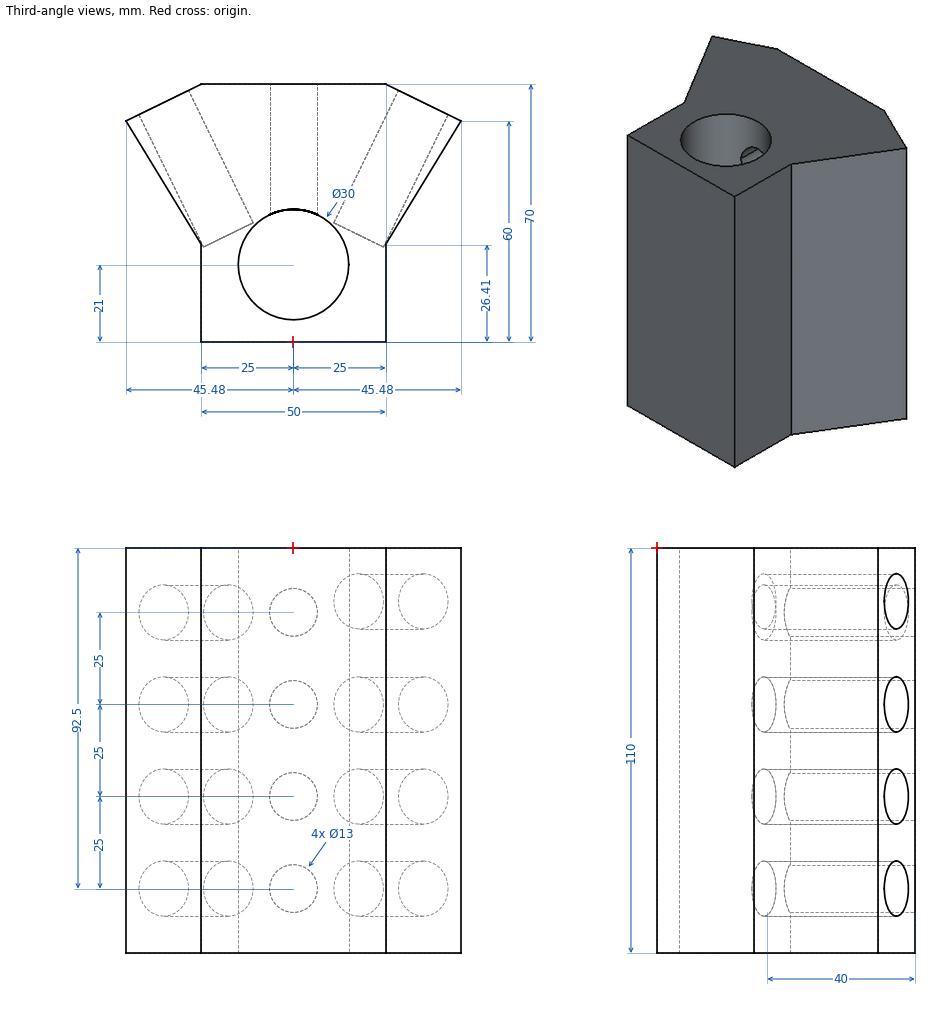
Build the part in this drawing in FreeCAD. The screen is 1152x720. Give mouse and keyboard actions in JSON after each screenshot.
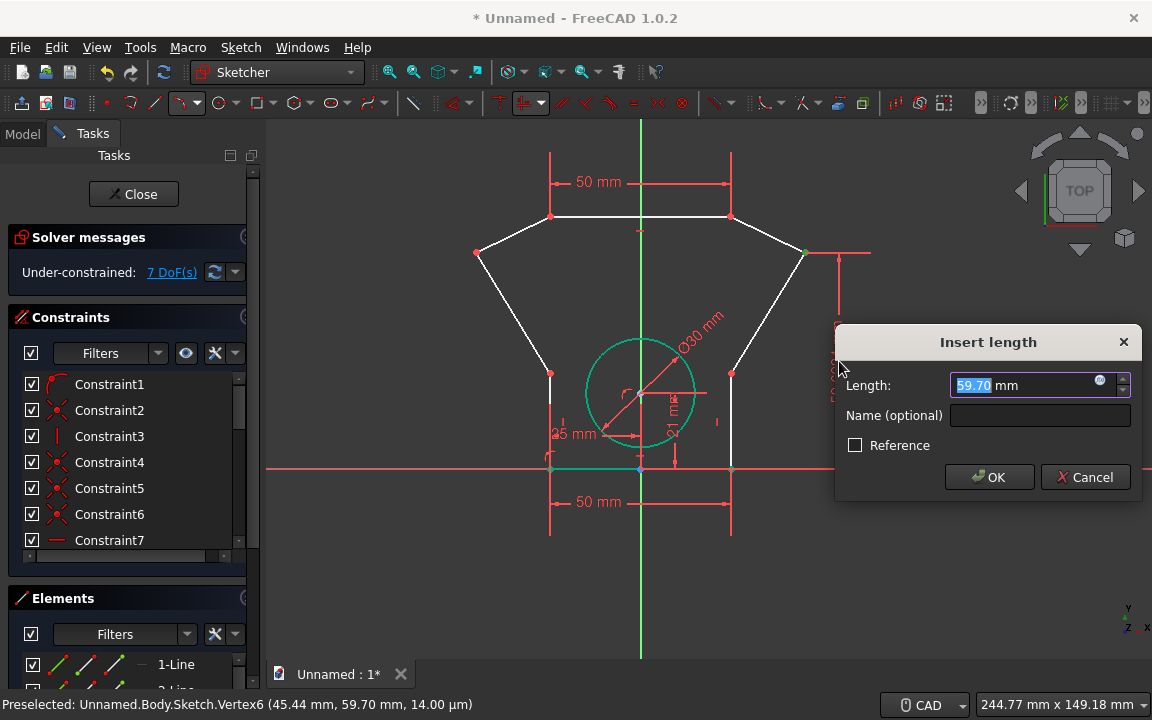
{"action": "type", "text": "60"}
{"action": "key", "text": "Return"}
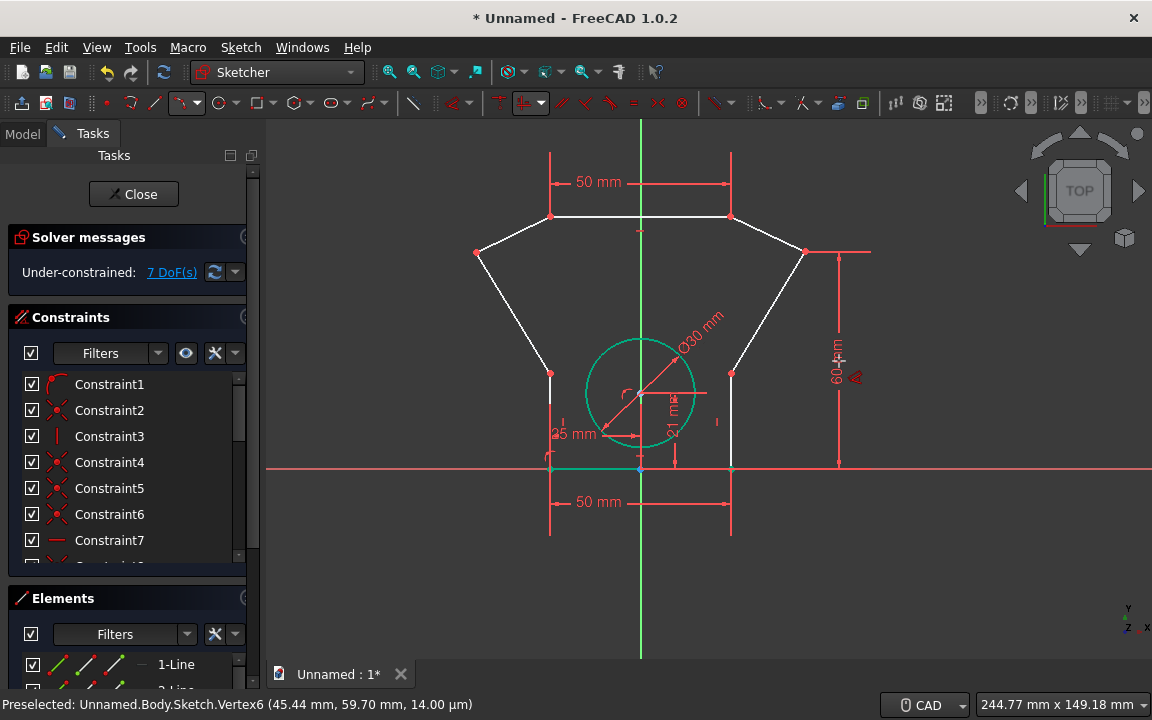
{"action": "left_click", "coordinate": [731, 217]}
{"action": "left_click", "coordinate": [686, 503]}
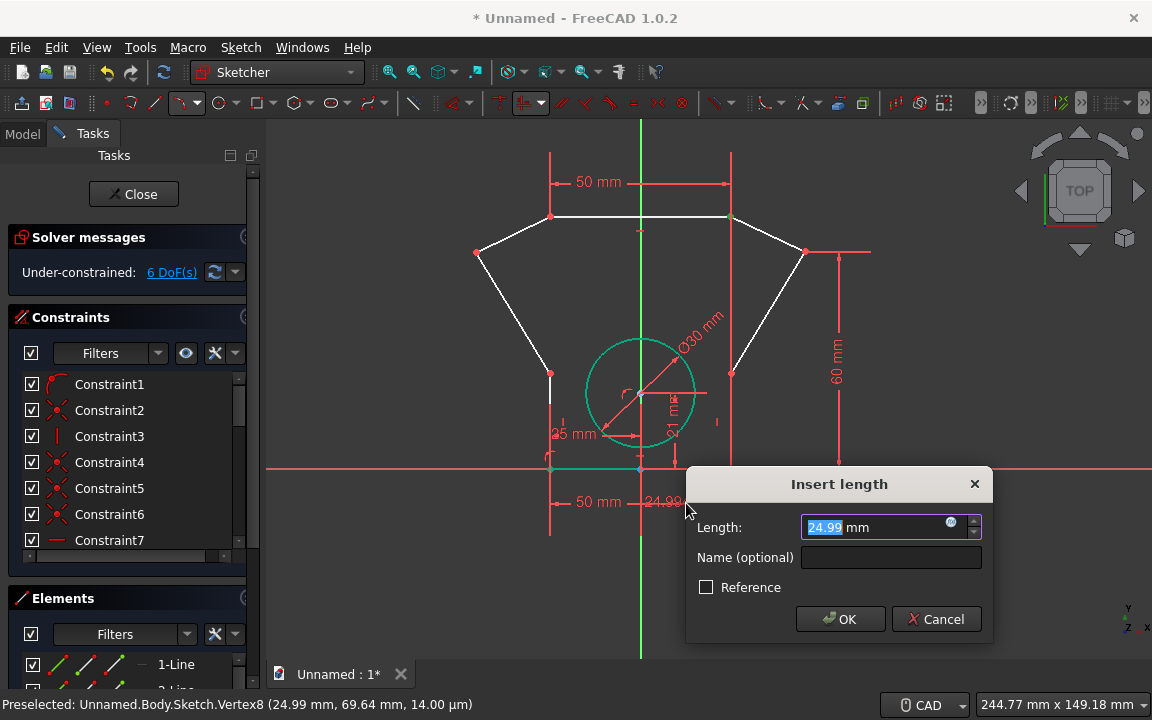
{"action": "type", "text": "25"}
{"action": "key", "text": "Return"}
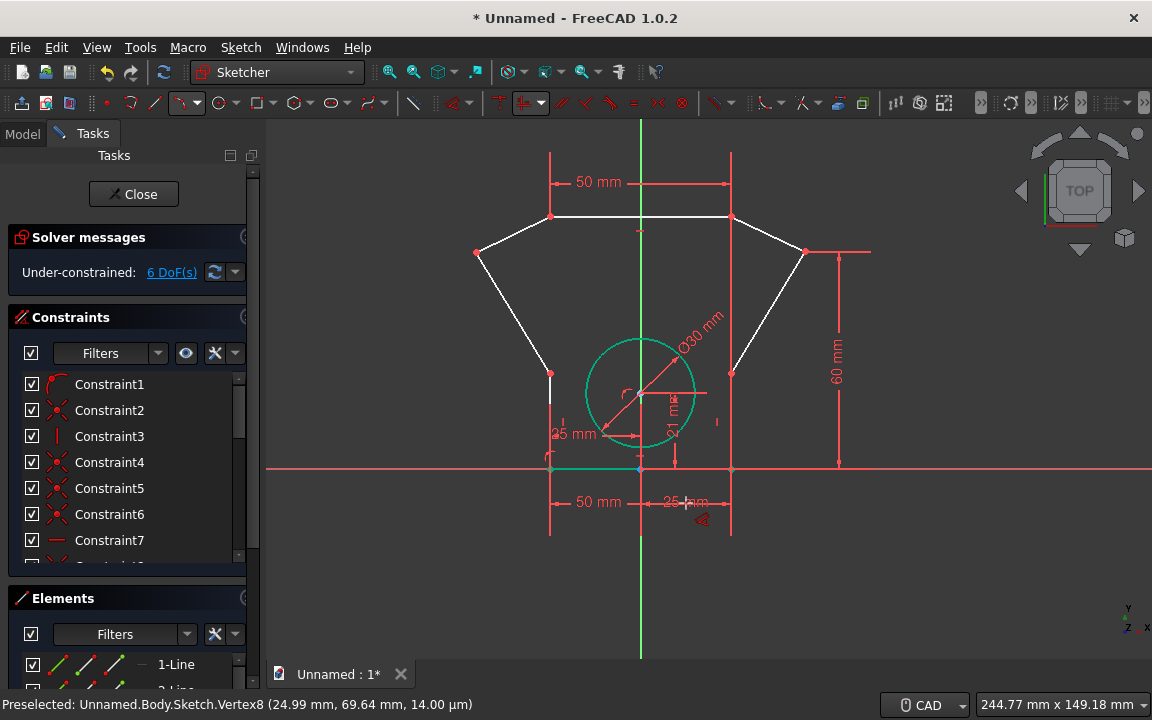
{"action": "left_click", "coordinate": [731, 217]}
{"action": "left_click", "coordinate": [765, 285]}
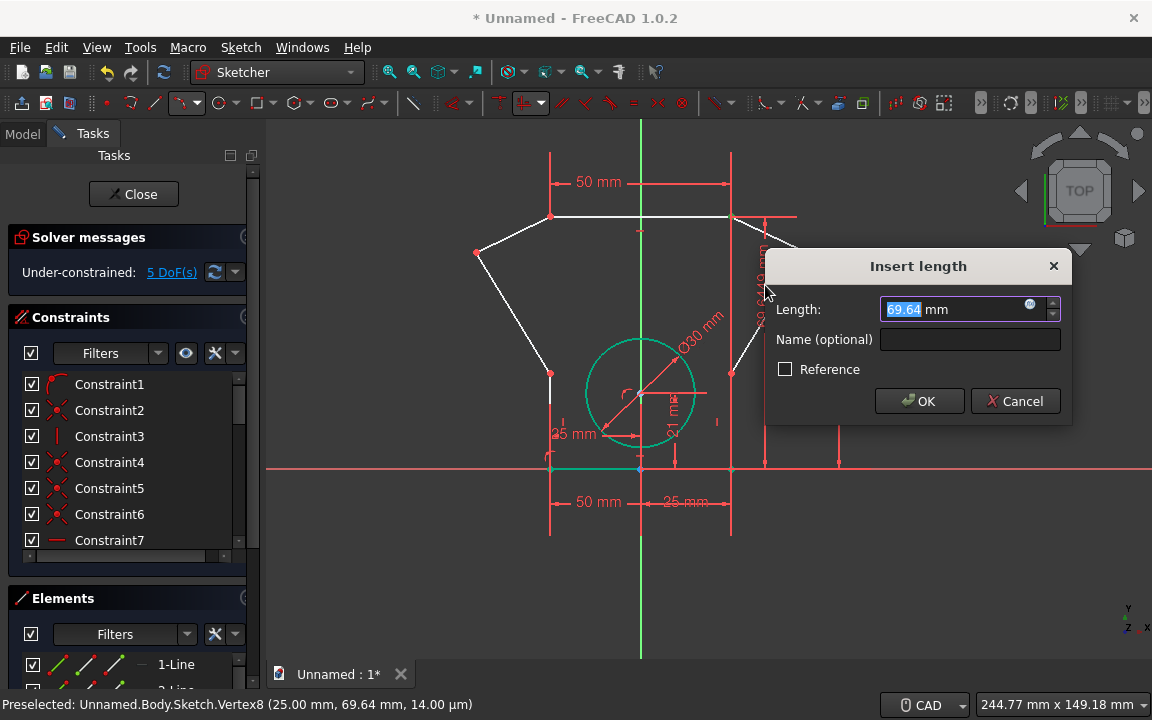
{"action": "type", "text": "70"}
{"action": "key", "text": "Return"}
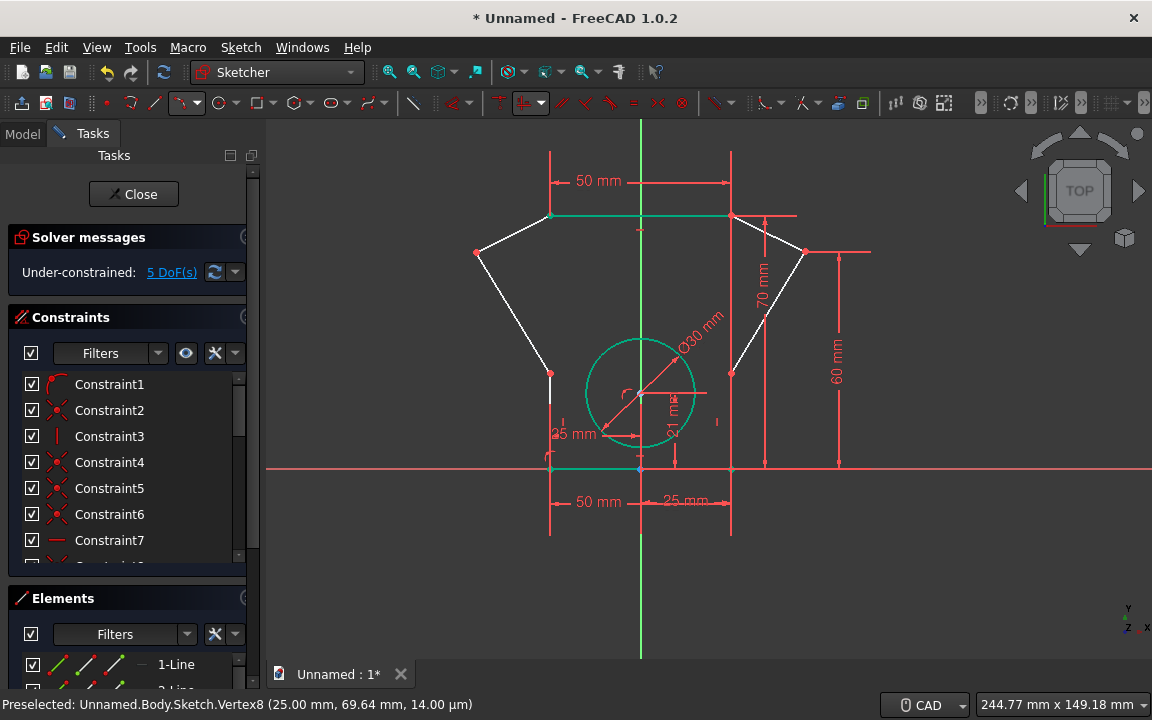
{"action": "left_click", "coordinate": [476, 253]}
{"action": "left_click", "coordinate": [442, 361]}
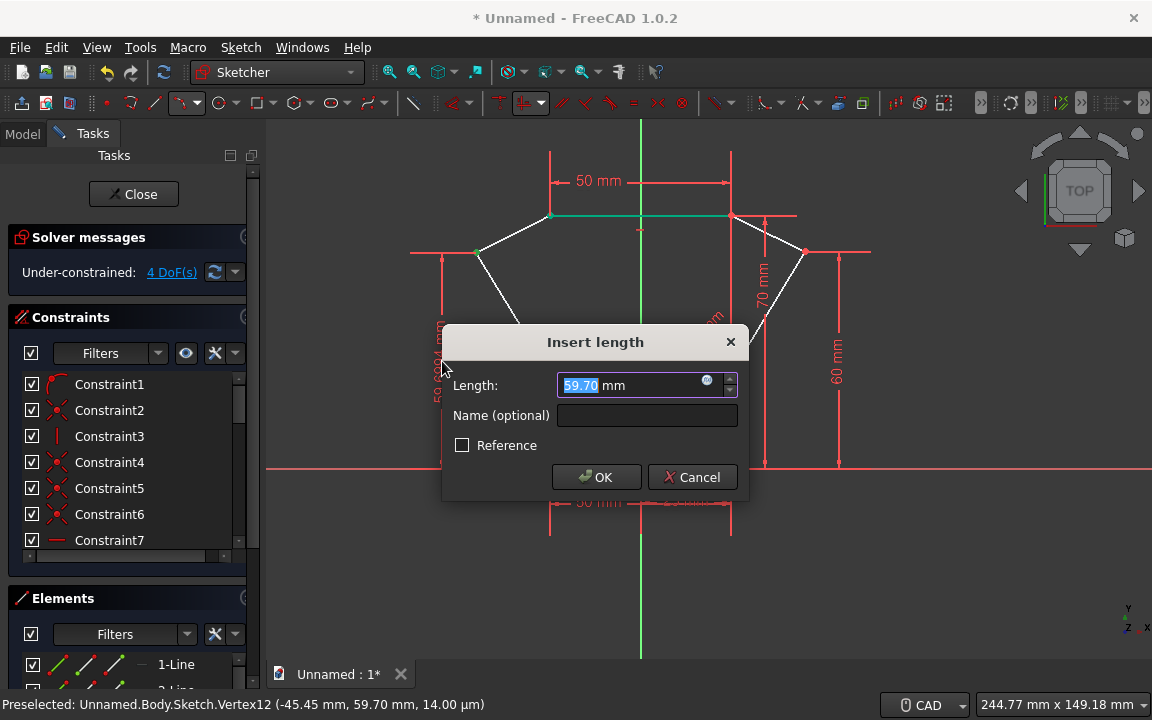
{"action": "type", "text": "60"}
{"action": "key", "text": "Return"}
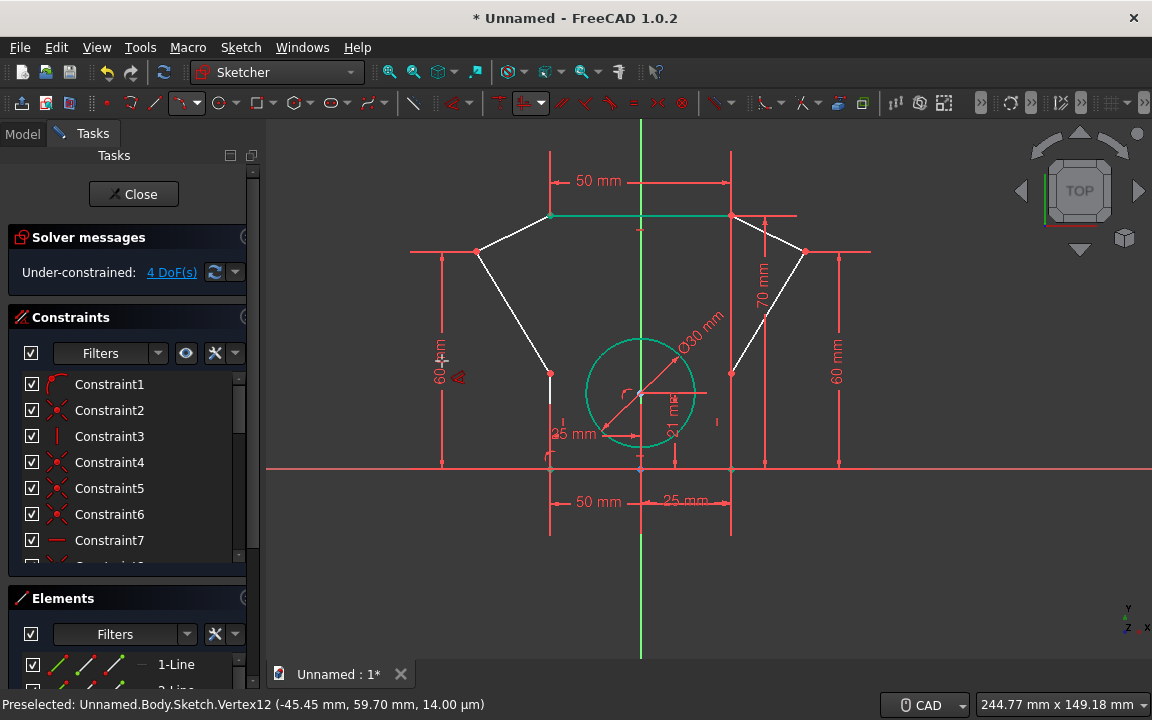
{"action": "left_click", "coordinate": [731, 441]}
{"action": "left_click", "coordinate": [765, 422]}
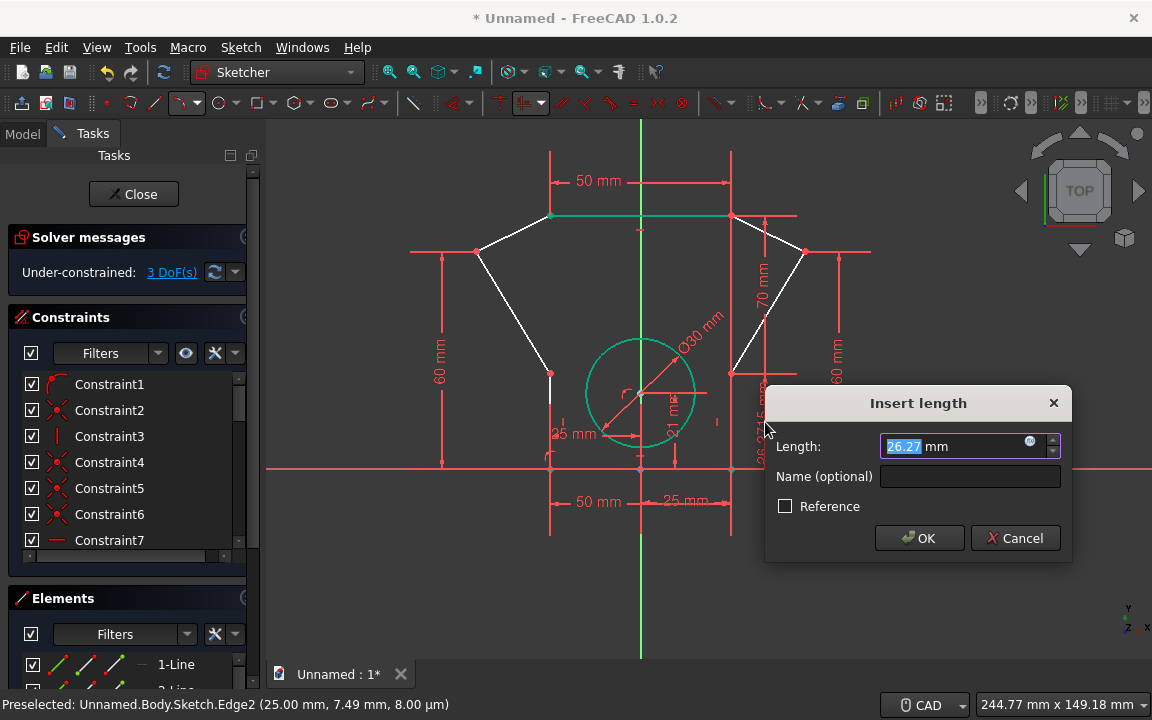
{"action": "type", "text": "26.41"}
{"action": "key", "text": "Return"}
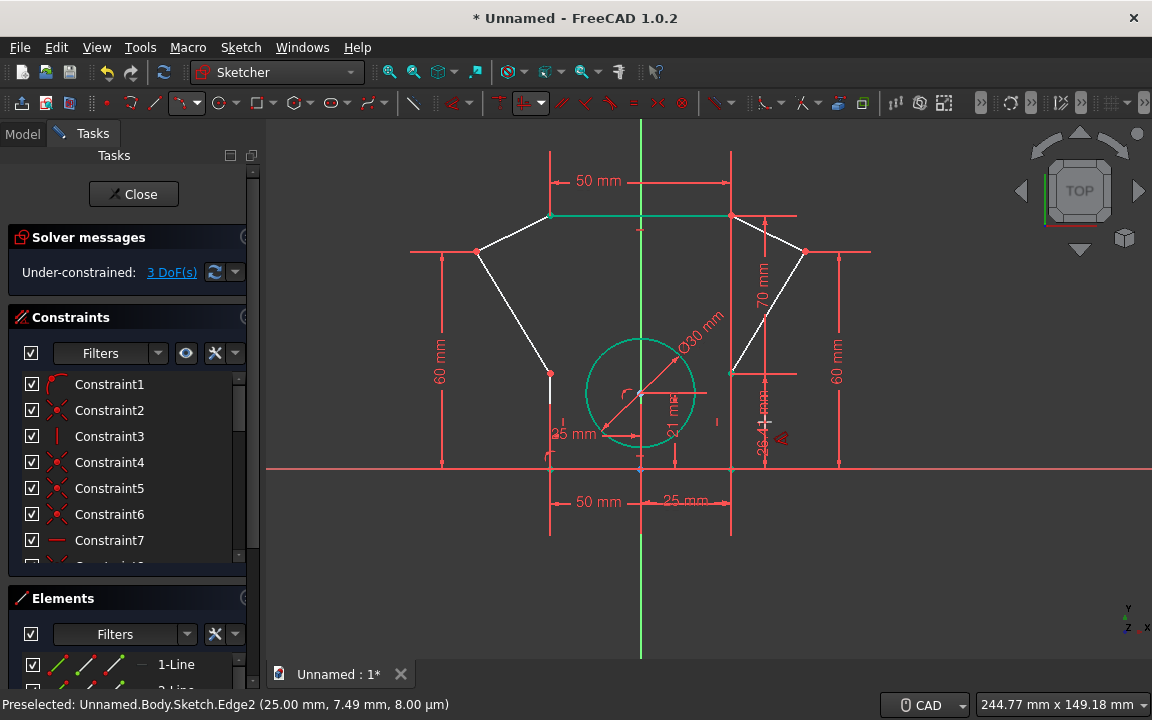
{"action": "left_click", "coordinate": [550, 403]}
{"action": "left_click", "coordinate": [516, 400]}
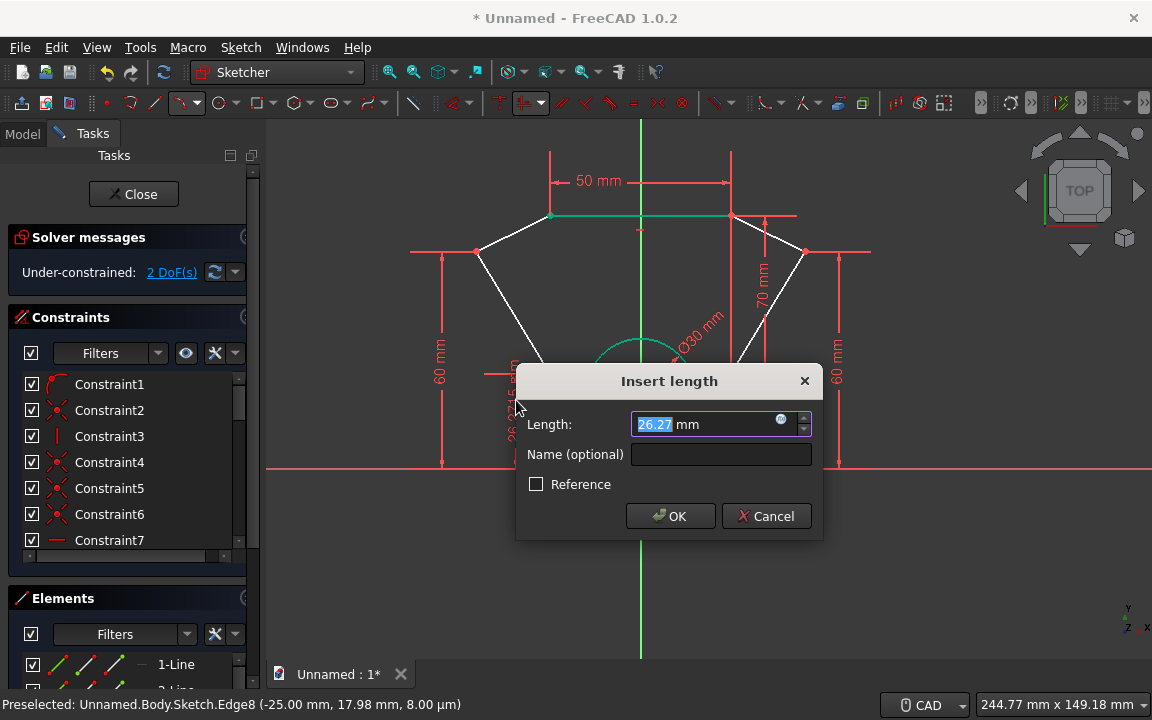
{"action": "type", "text": "26.41"}
{"action": "key", "text": "Return"}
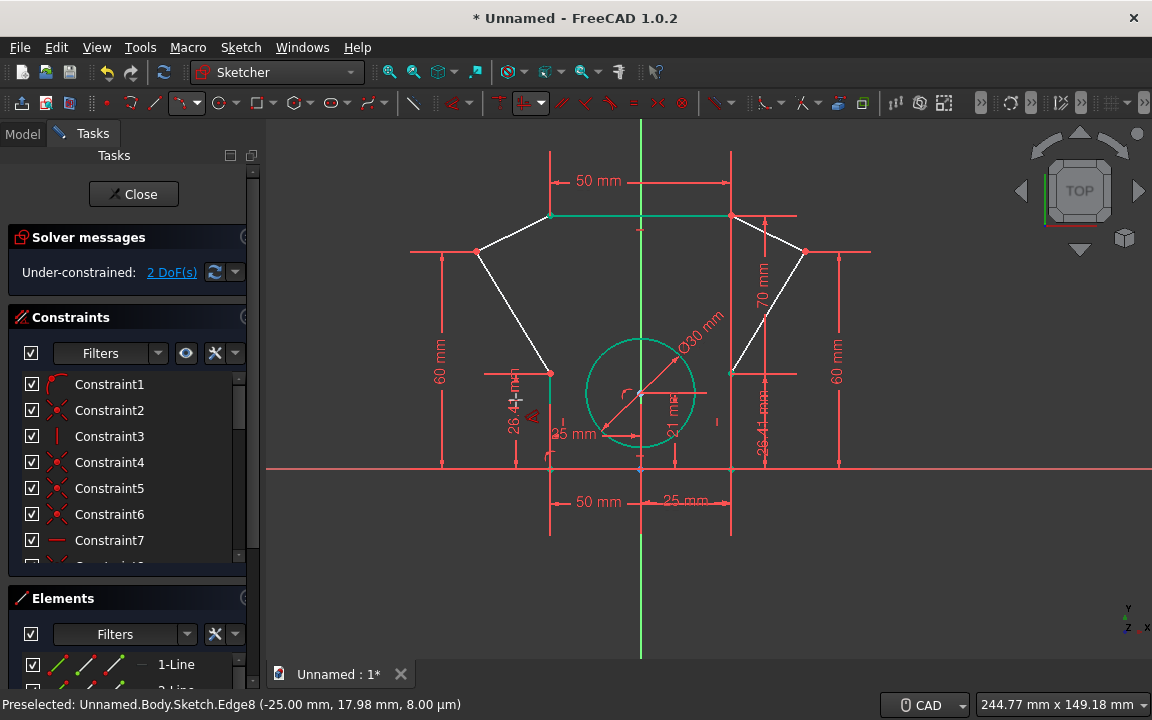
{"action": "left_click", "coordinate": [805, 252]}
{"action": "left_click", "coordinate": [761, 503]}